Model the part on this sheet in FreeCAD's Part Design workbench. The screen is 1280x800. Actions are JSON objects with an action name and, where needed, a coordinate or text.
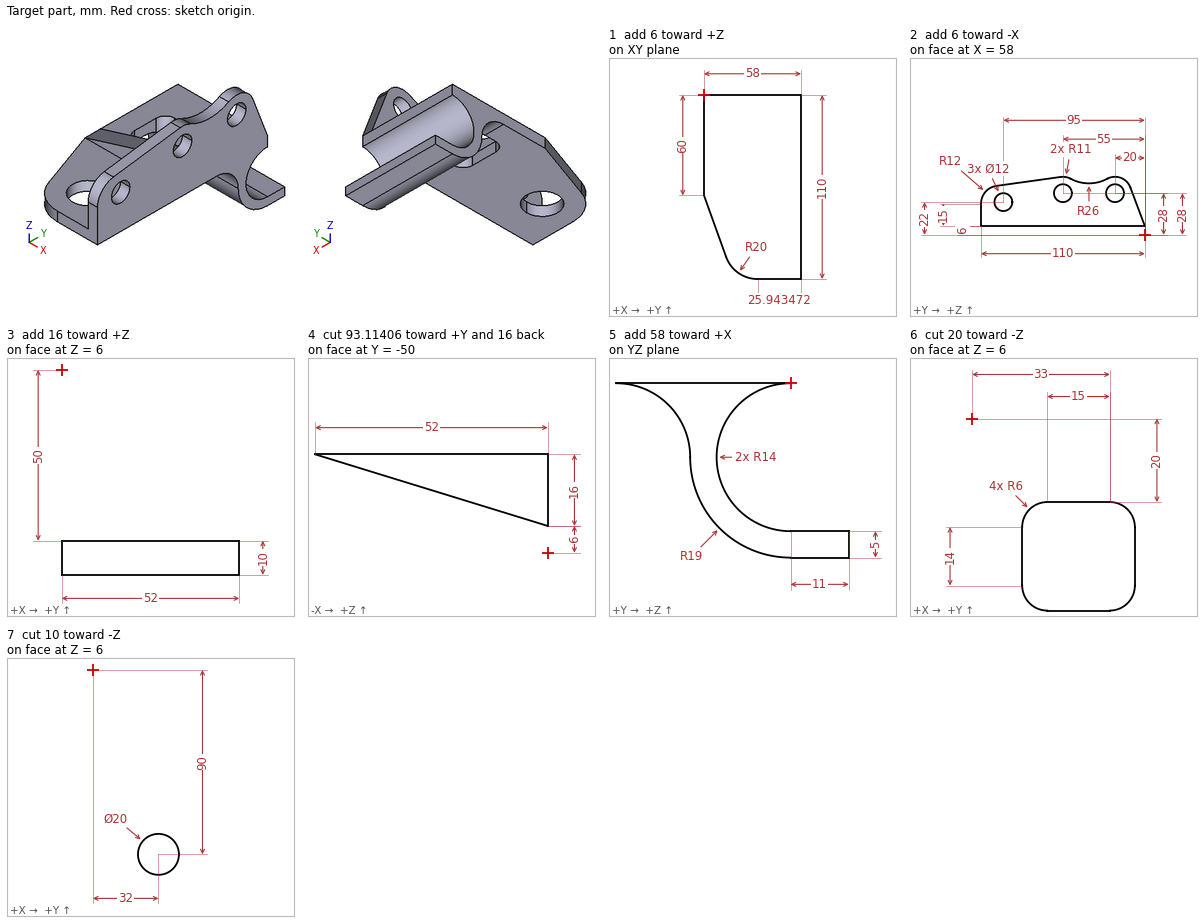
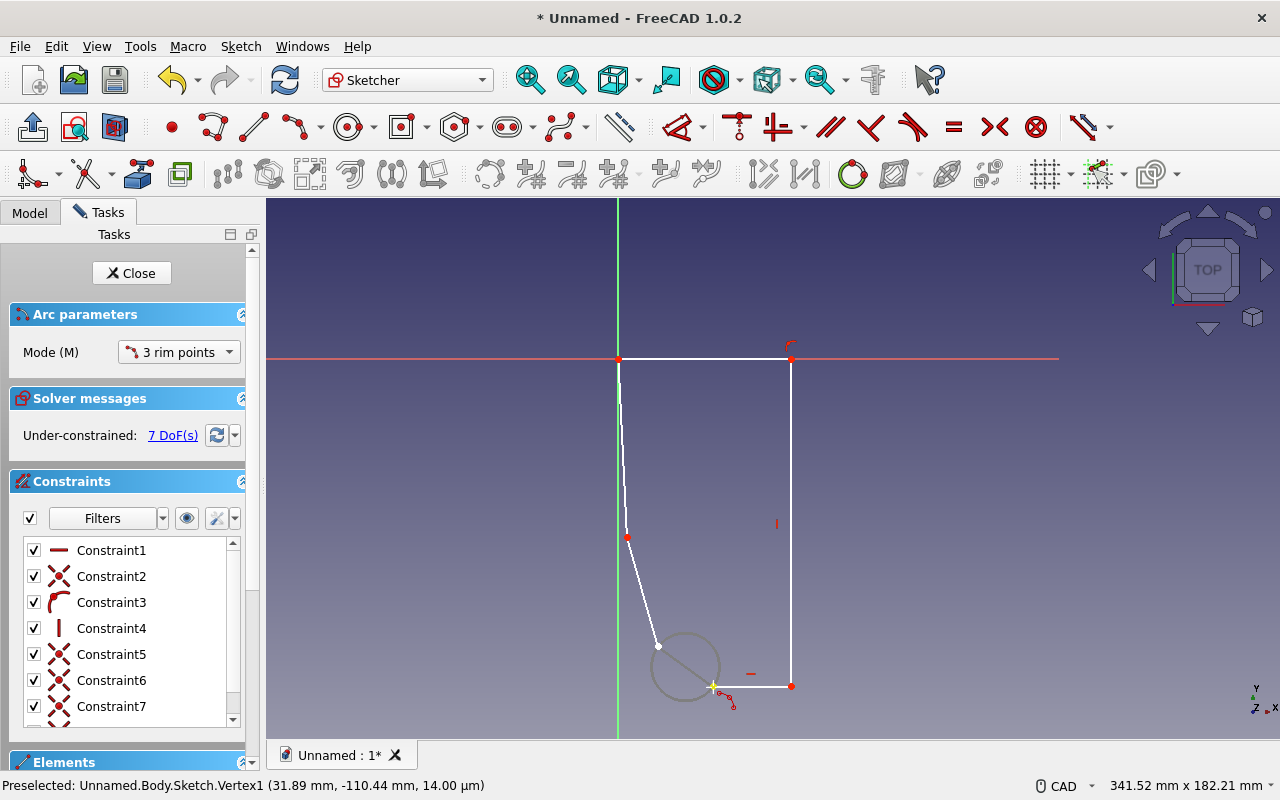
{"action": "scroll", "coordinate": [679, 675], "scroll_direction": "up", "scroll_amount": 2}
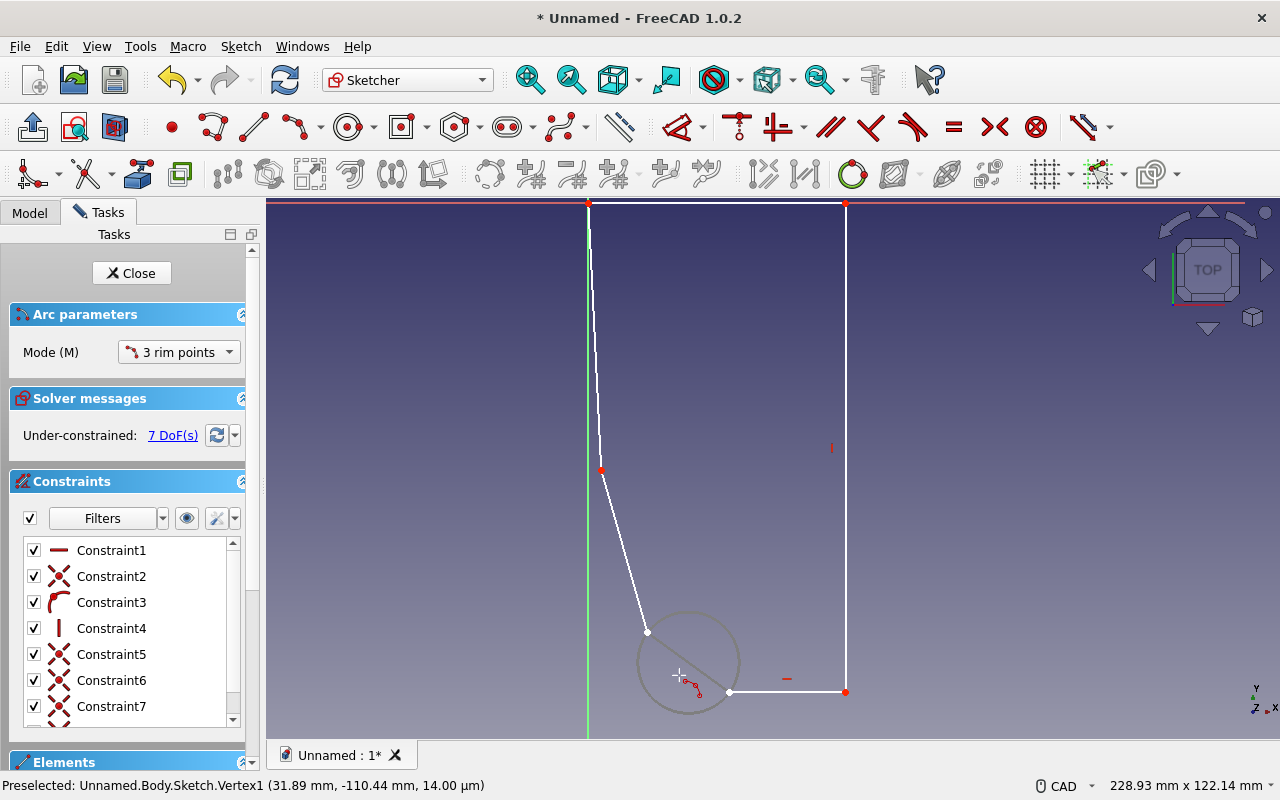
{"action": "left_click", "coordinate": [679, 674]}
{"action": "key", "text": "Escape"}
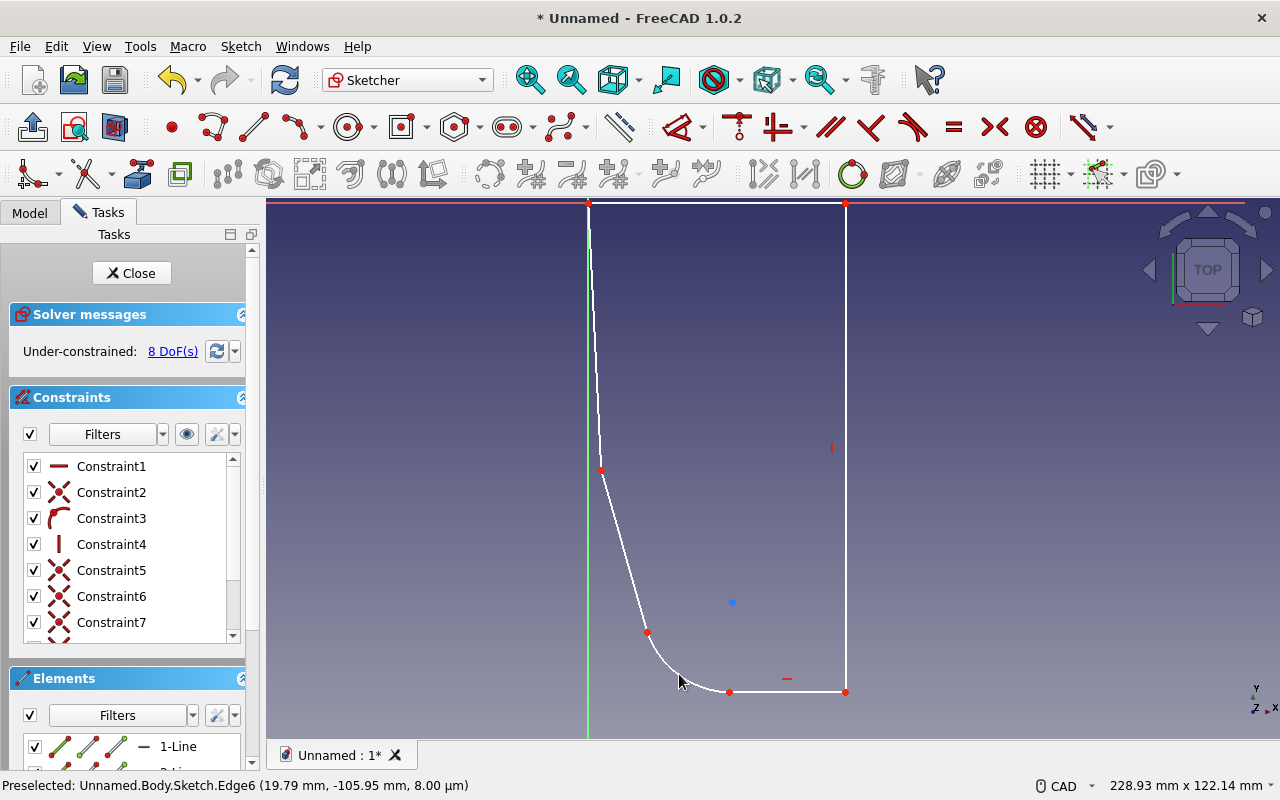
{"action": "left_click", "coordinate": [764, 692]}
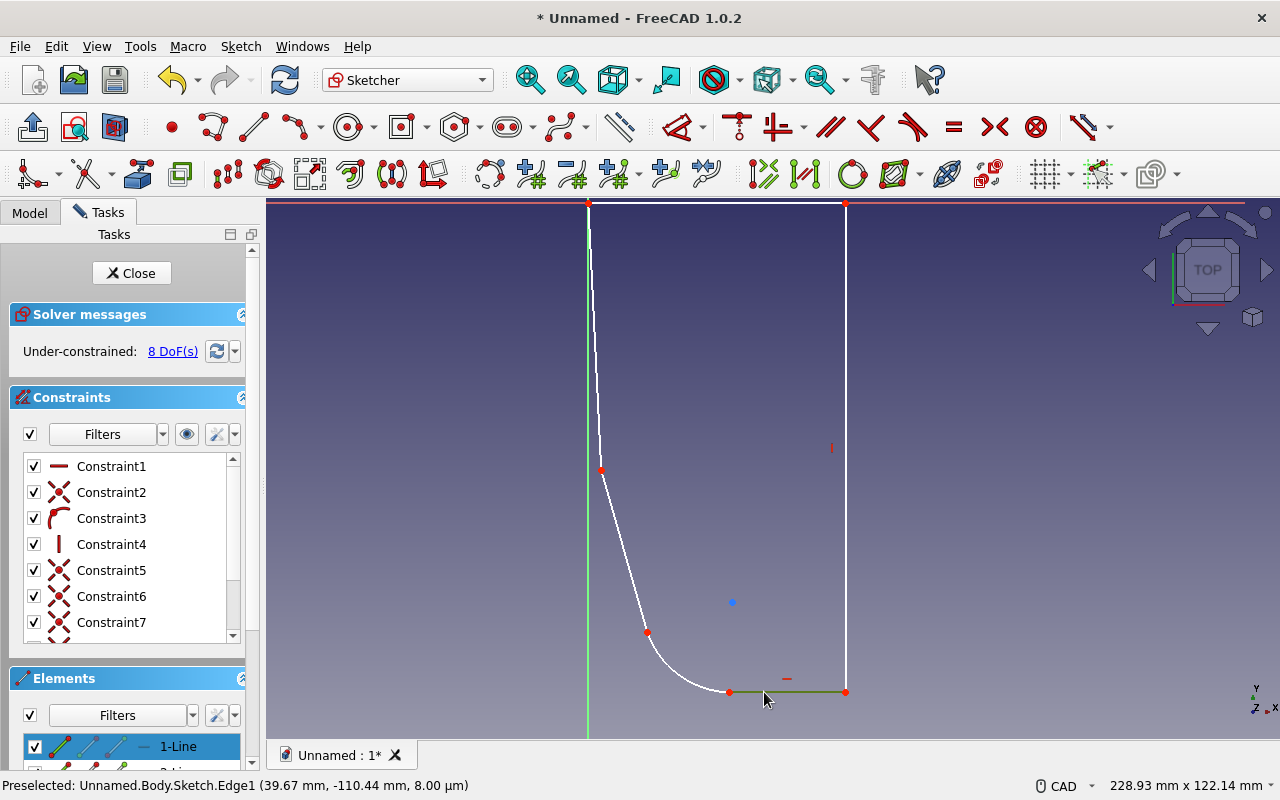
{"action": "left_click", "coordinate": [664, 661]}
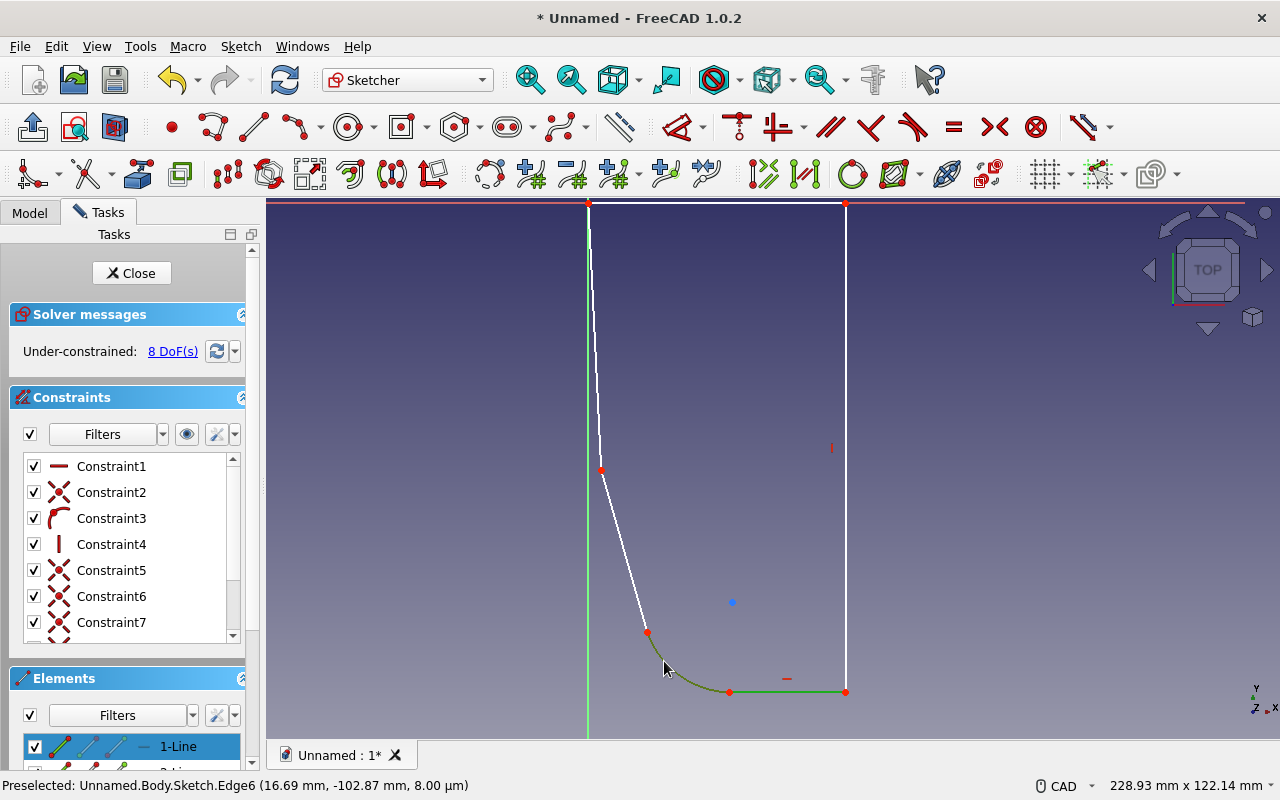
{"action": "left_click", "coordinate": [913, 128]}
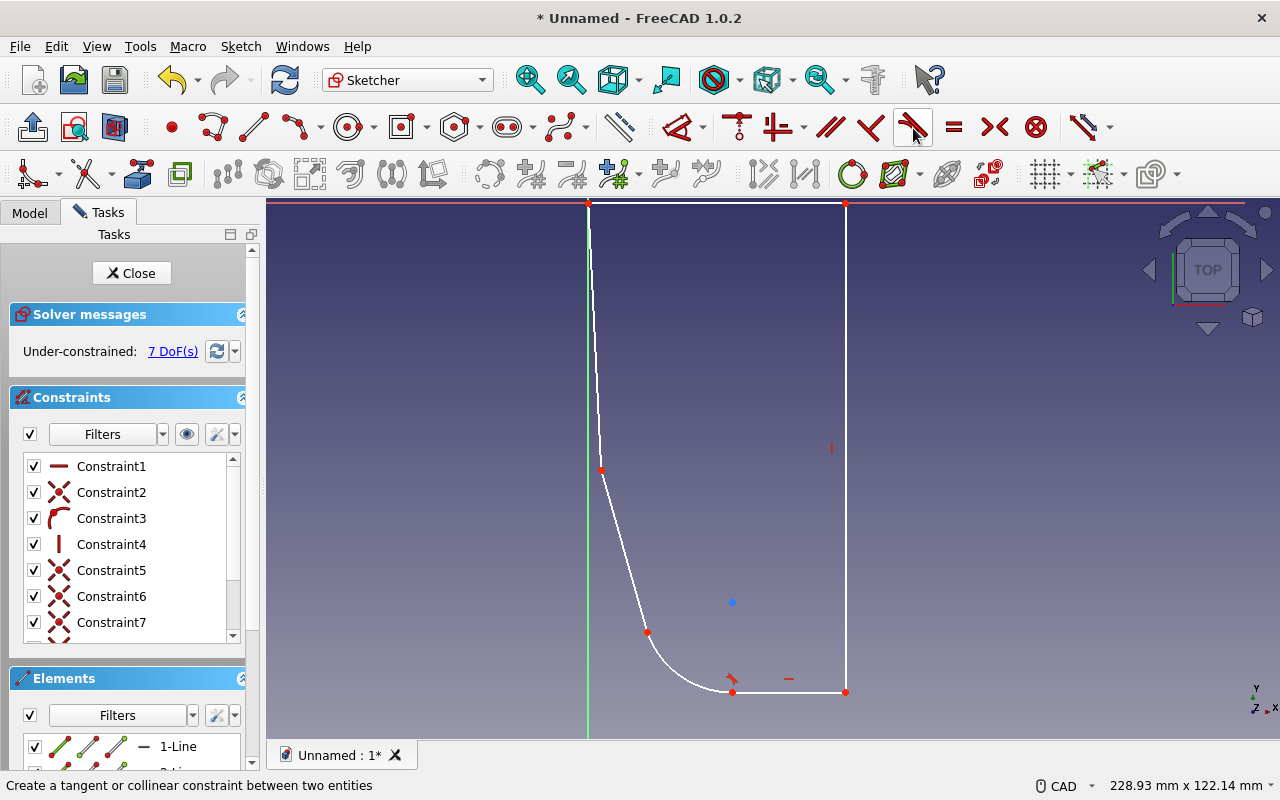
{"action": "left_click", "coordinate": [615, 519]}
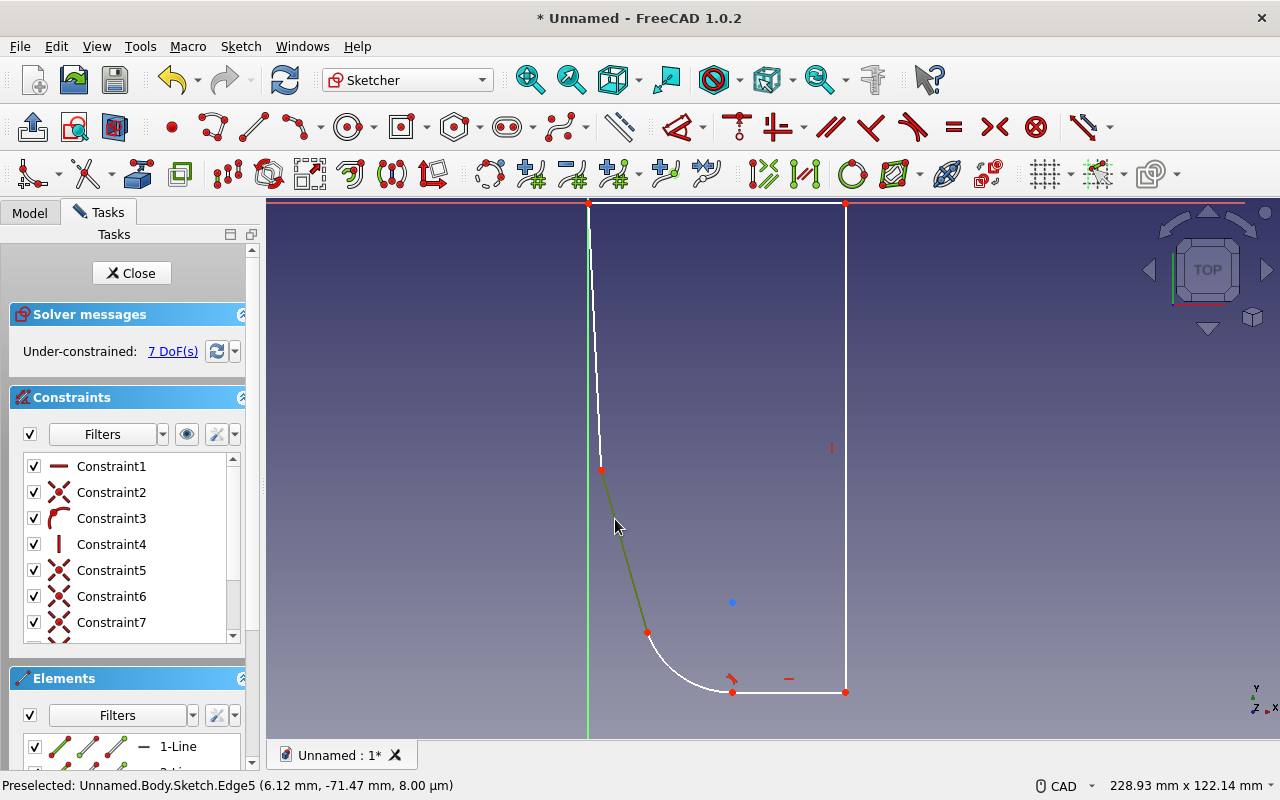
{"action": "left_click", "coordinate": [664, 661]}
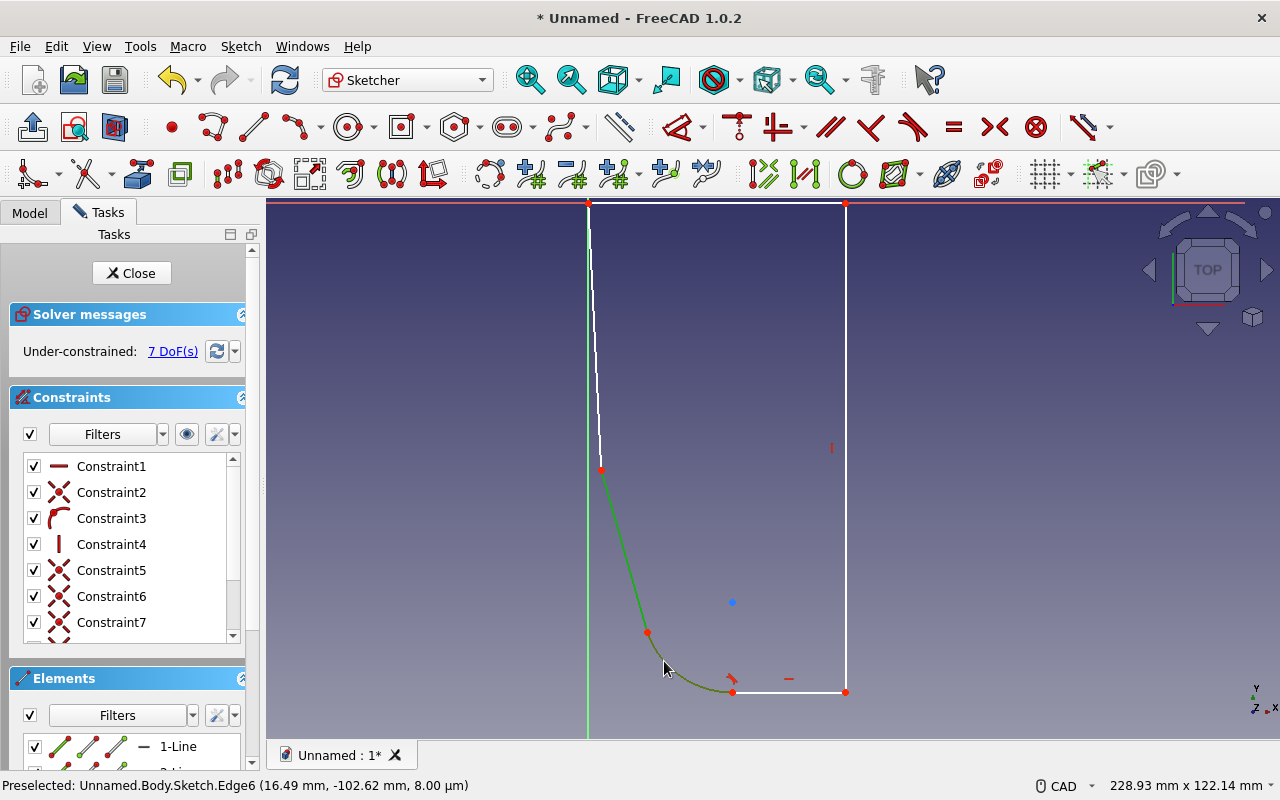
{"action": "left_click", "coordinate": [913, 128]}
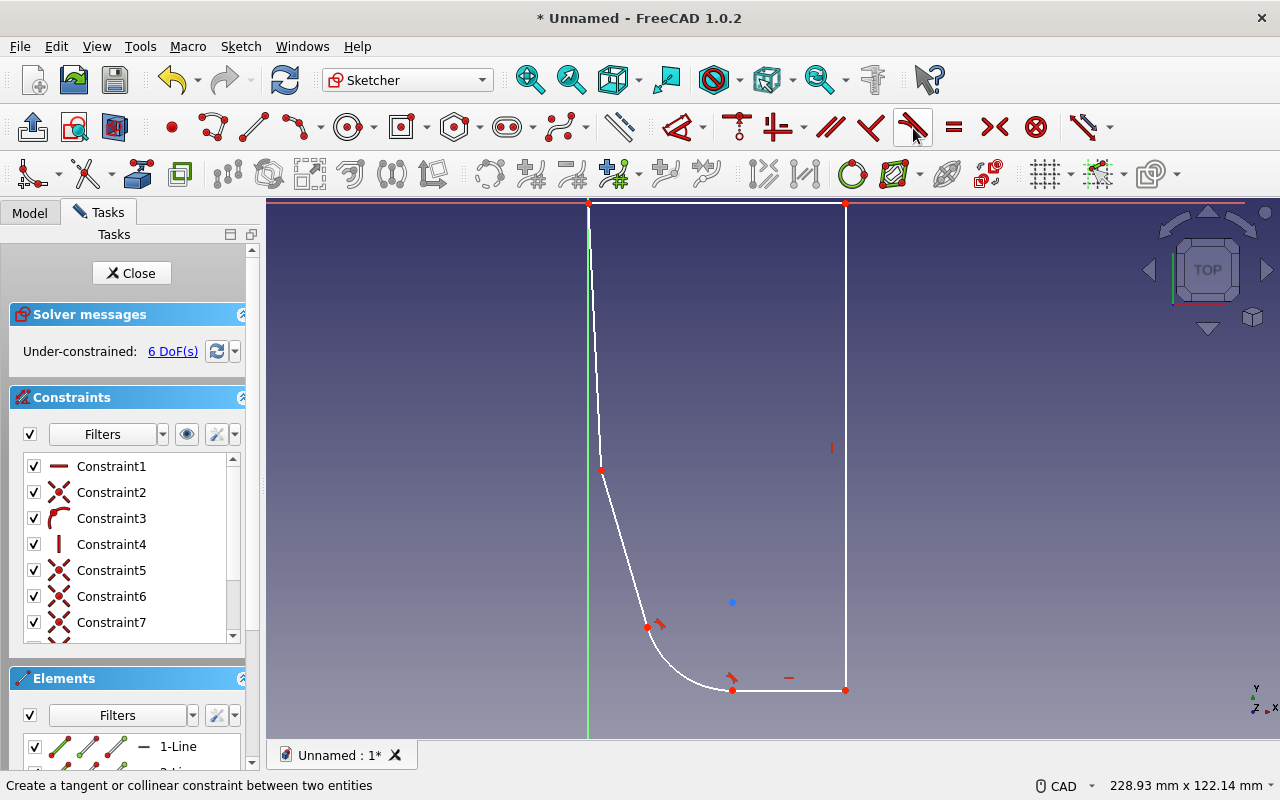
{"action": "left_click", "coordinate": [592, 283]}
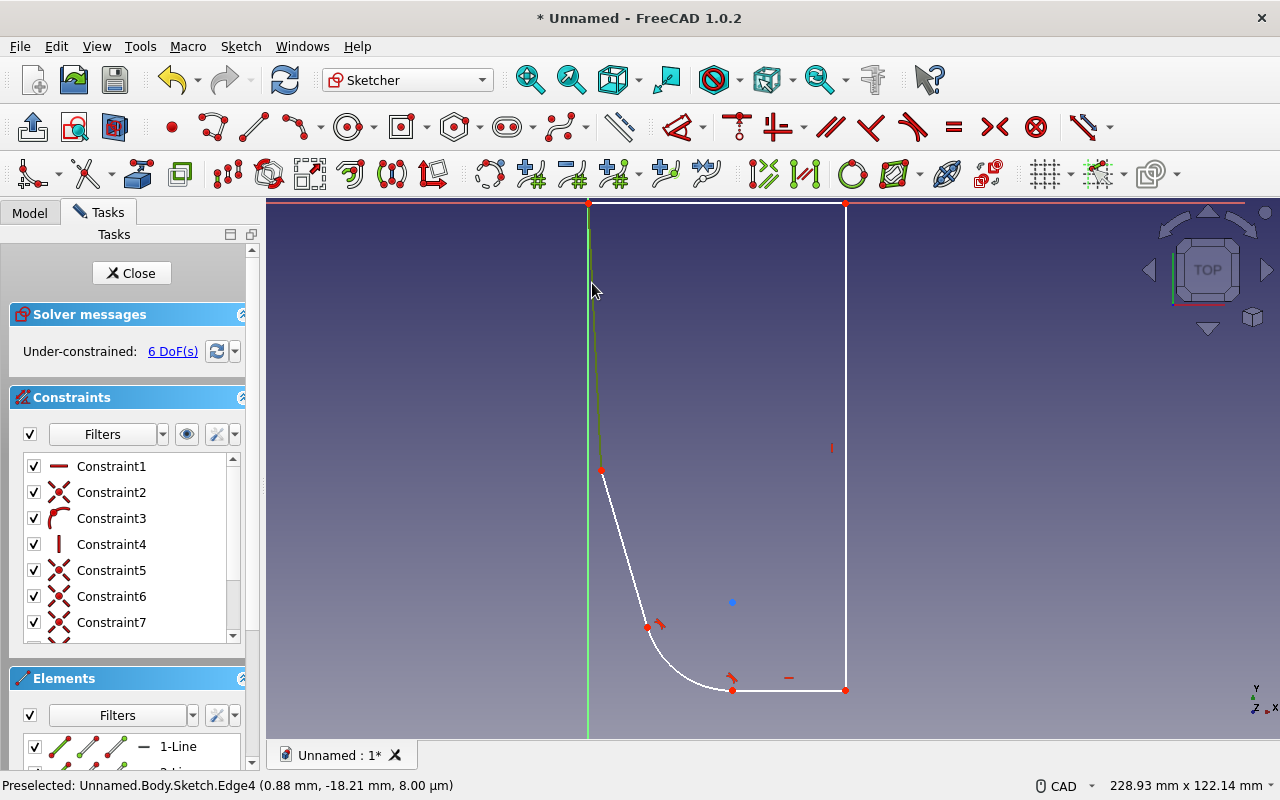
{"action": "left_click", "coordinate": [804, 128]}